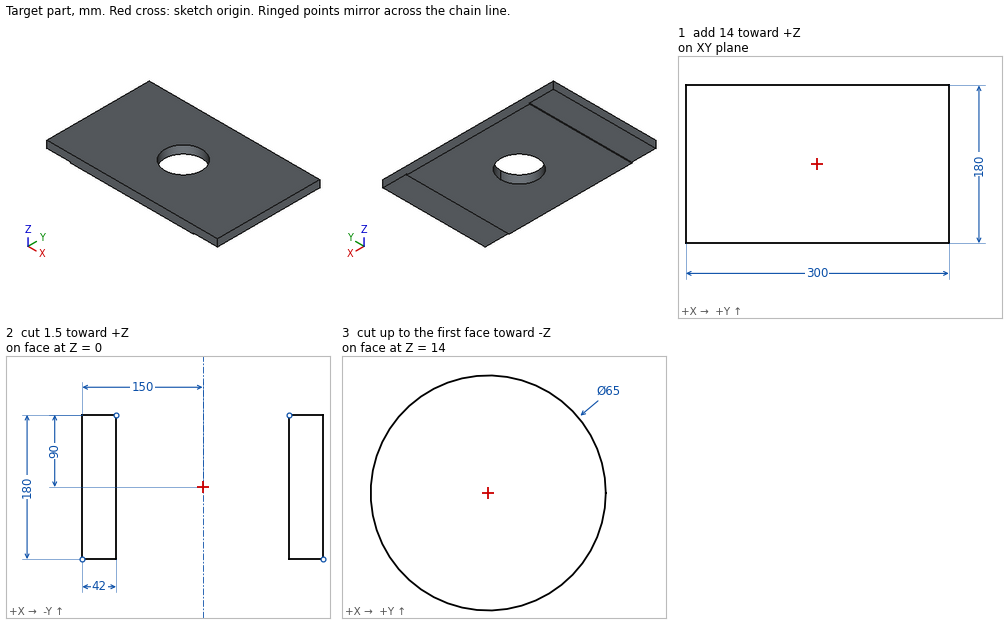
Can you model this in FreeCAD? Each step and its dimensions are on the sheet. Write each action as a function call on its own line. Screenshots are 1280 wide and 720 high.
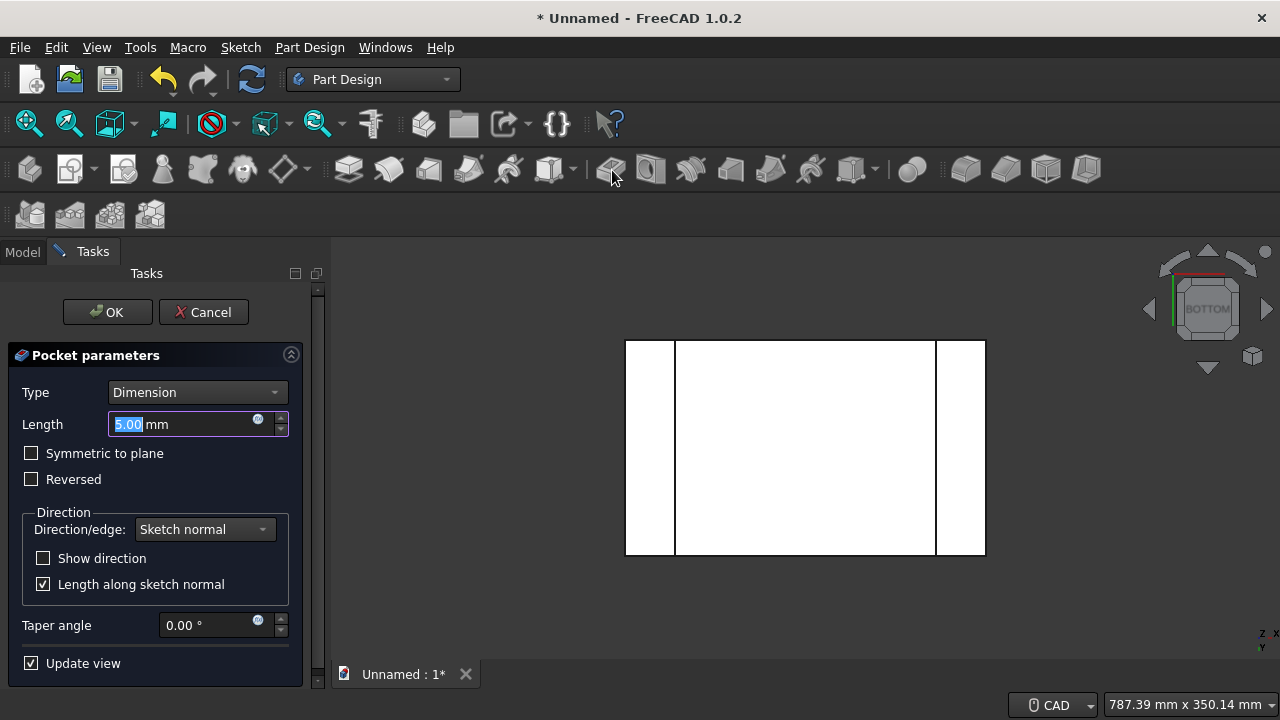
text(1.5)
key(Tab)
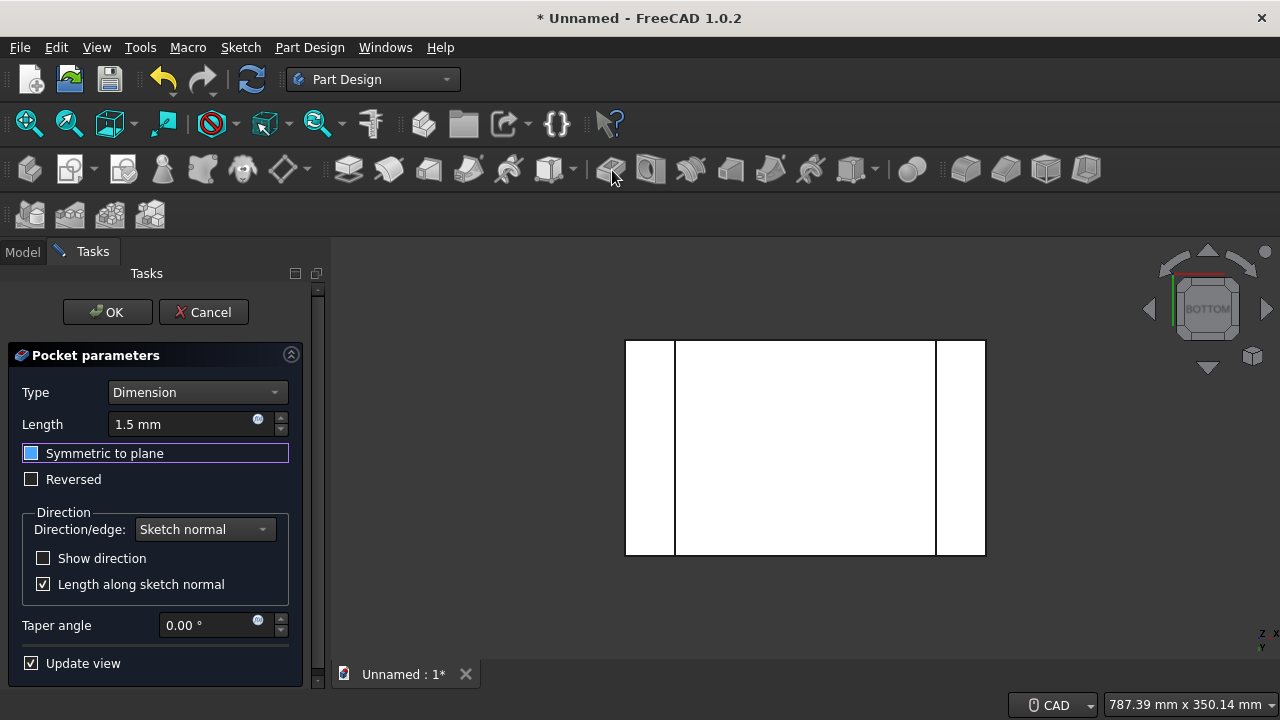
click(108, 312)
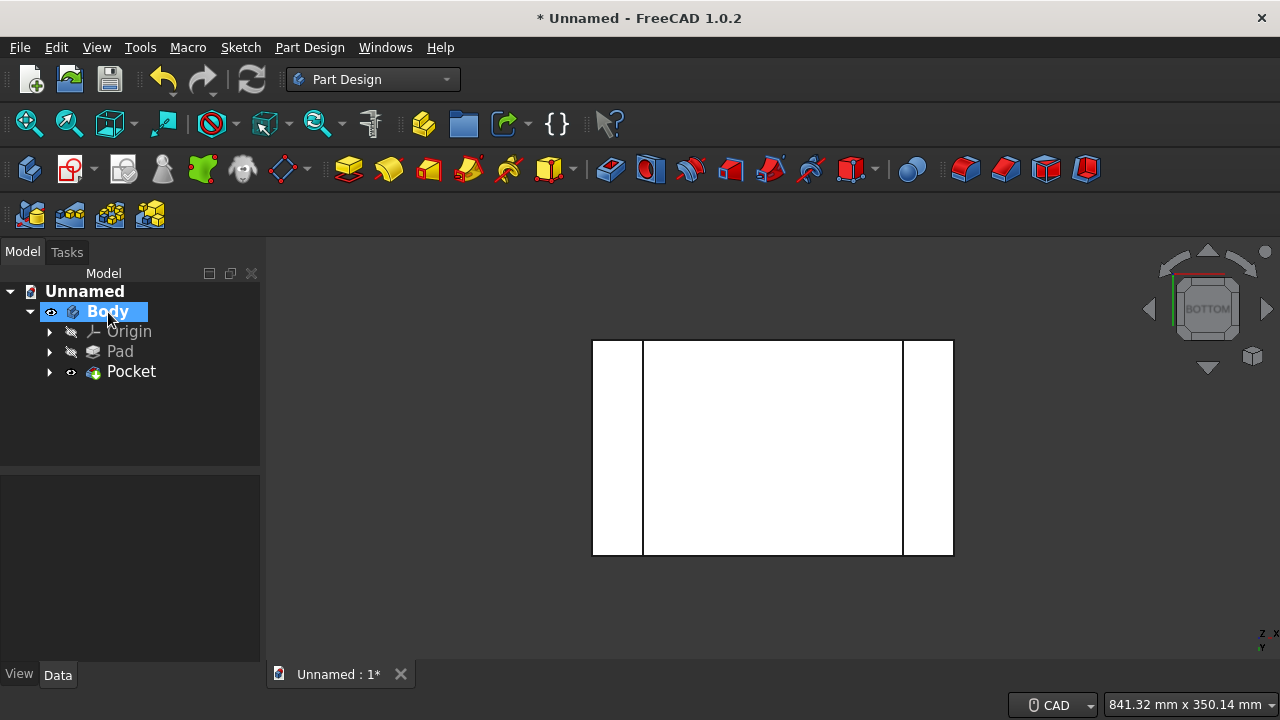
key(0)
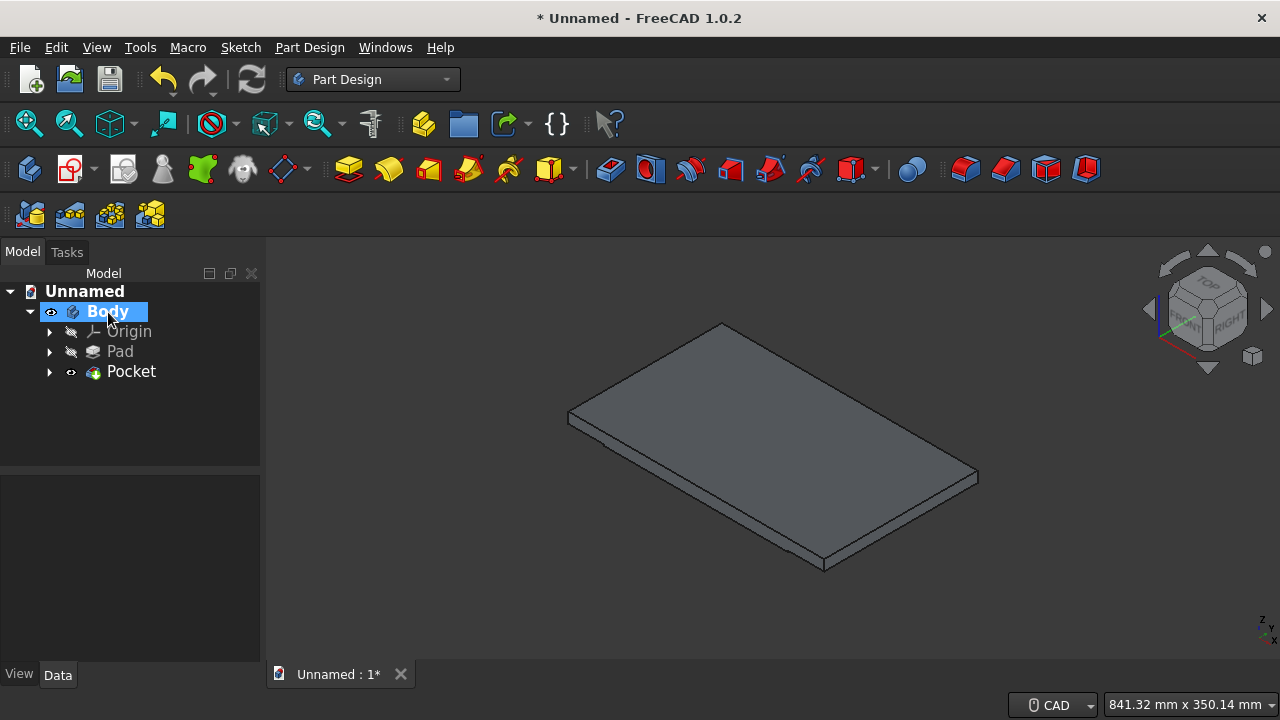
click(810, 461)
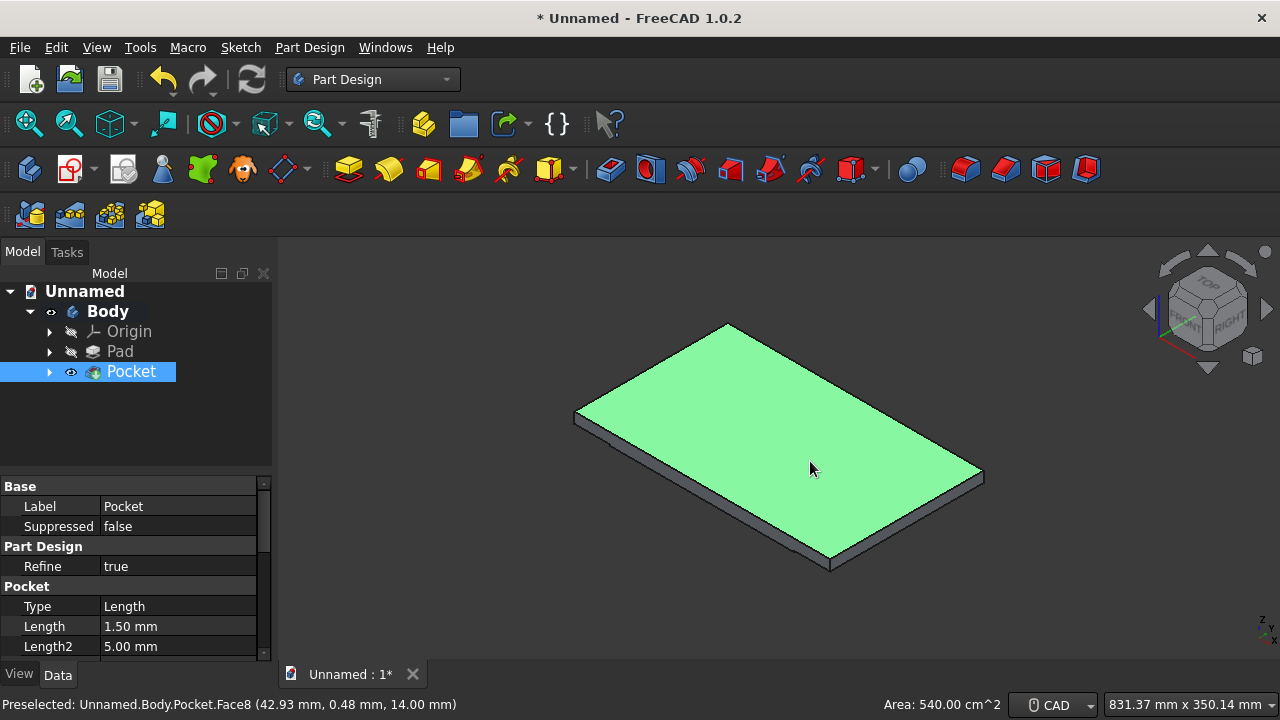
click(70, 170)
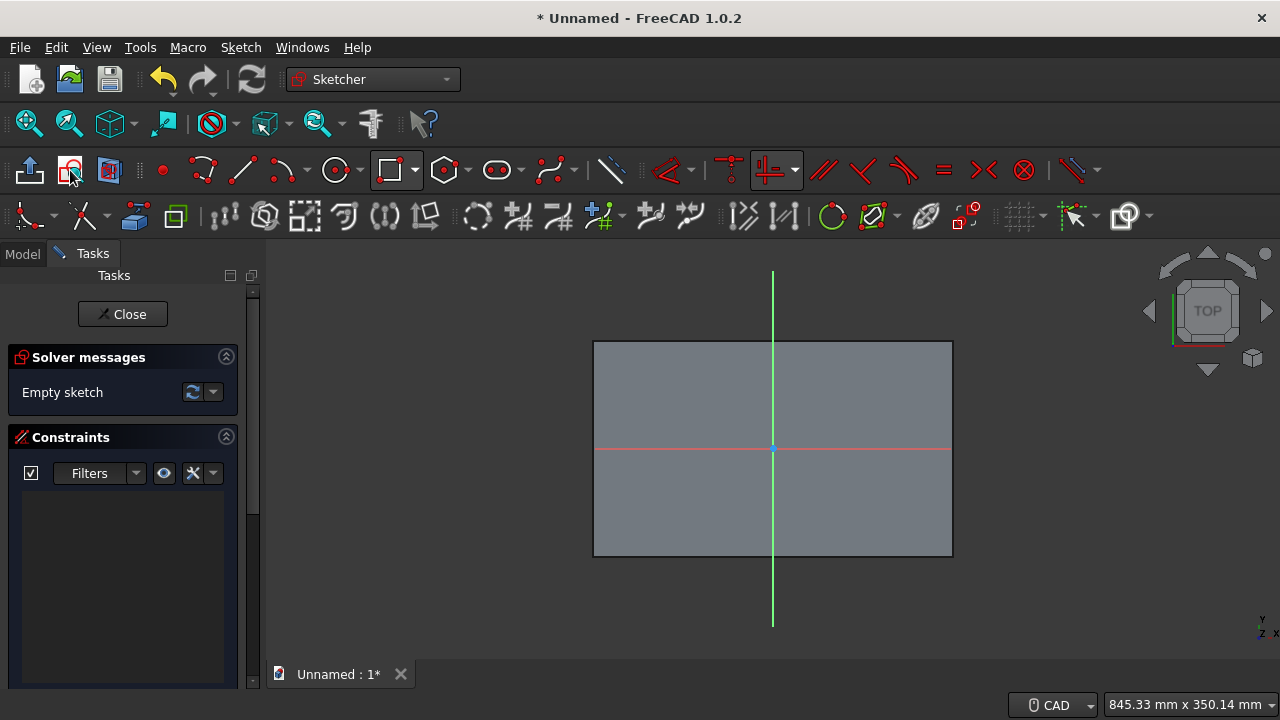
scroll(803, 449, up, 6)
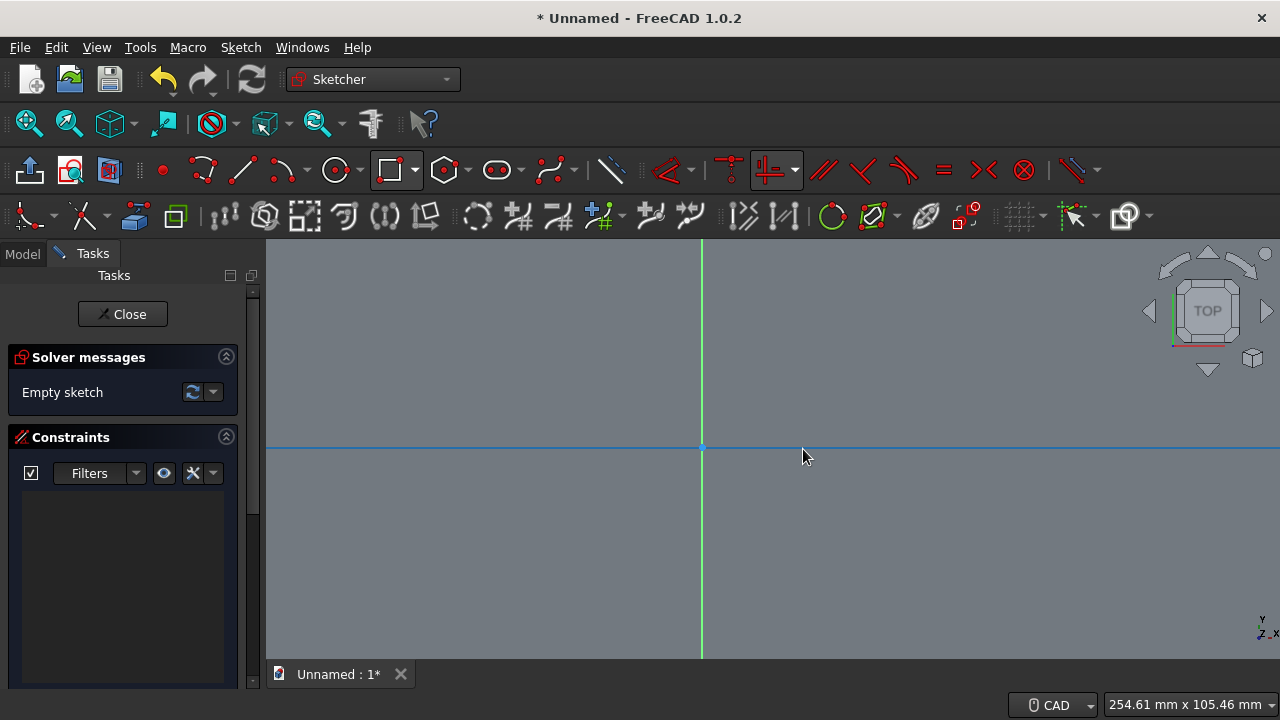
click(336, 170)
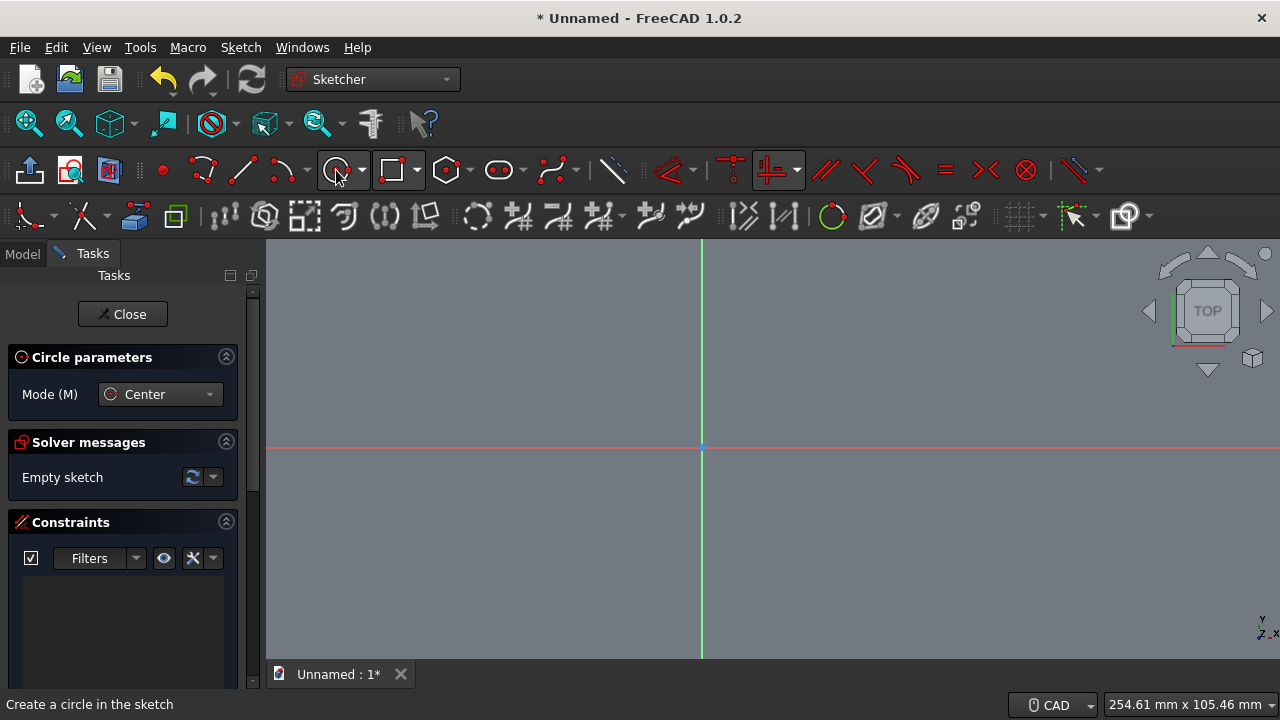
click(702, 448)
click(794, 356)
key(Escape)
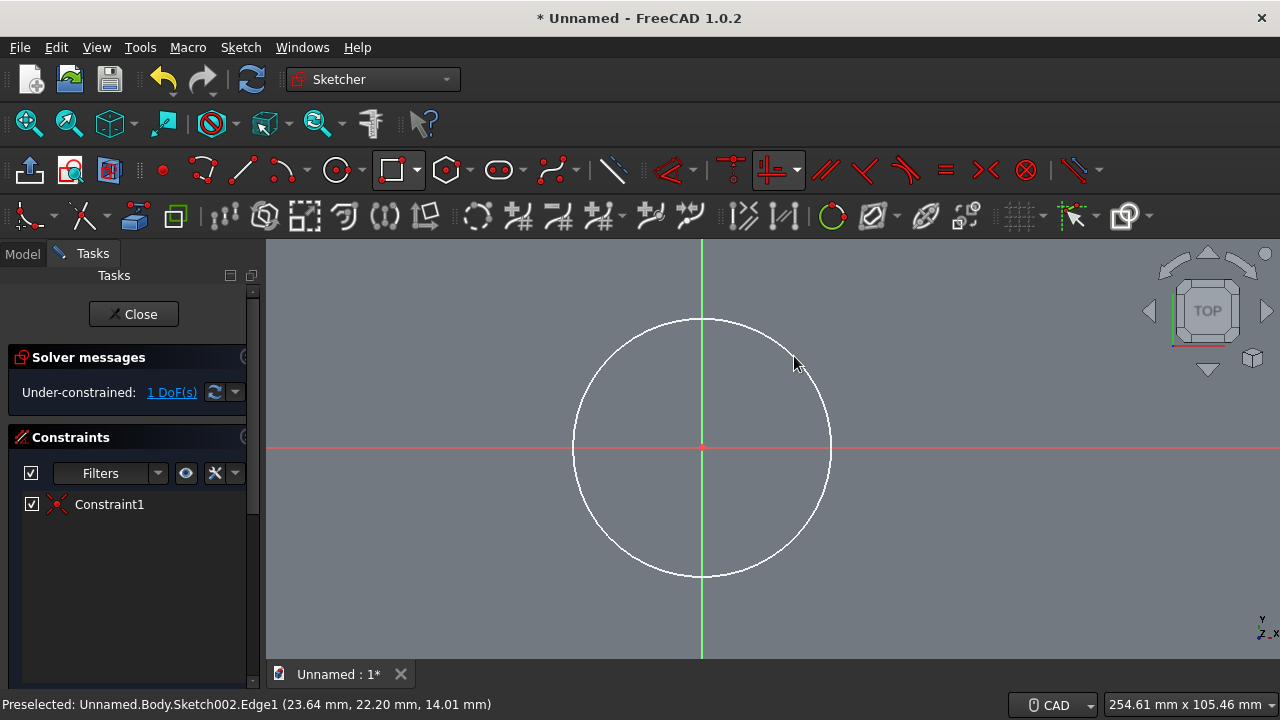
click(668, 170)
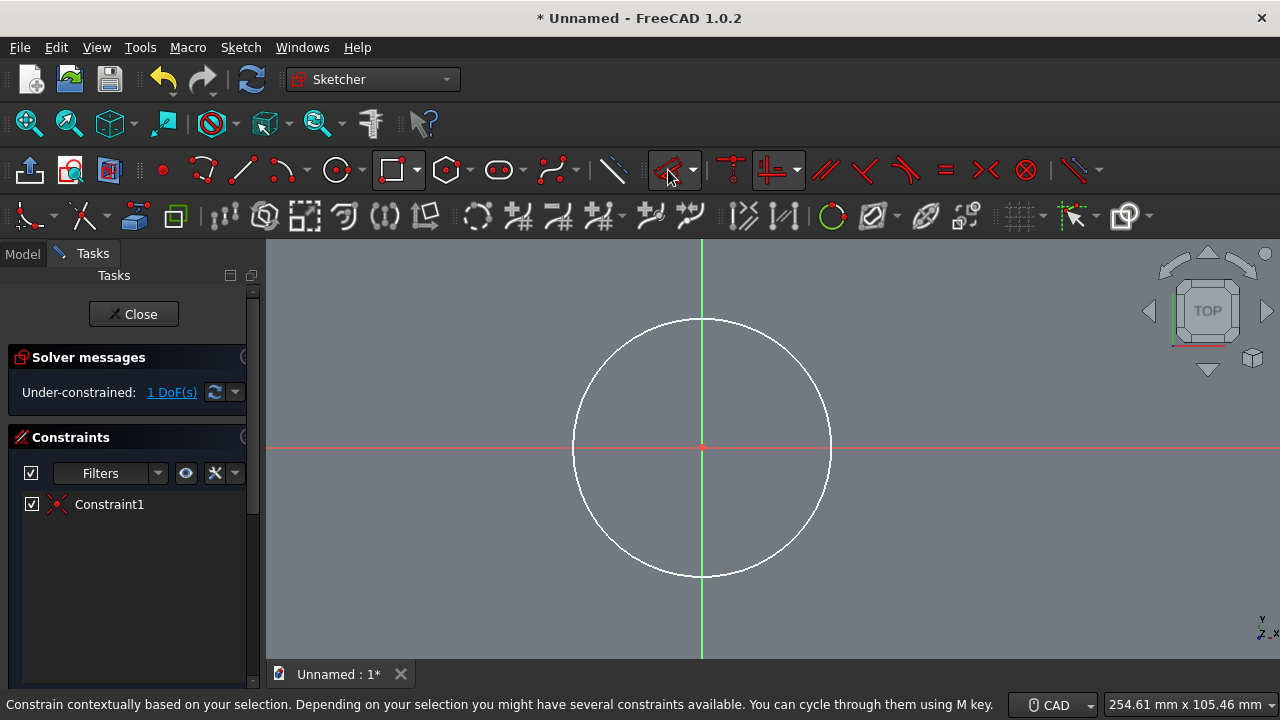
click(793, 356)
click(816, 333)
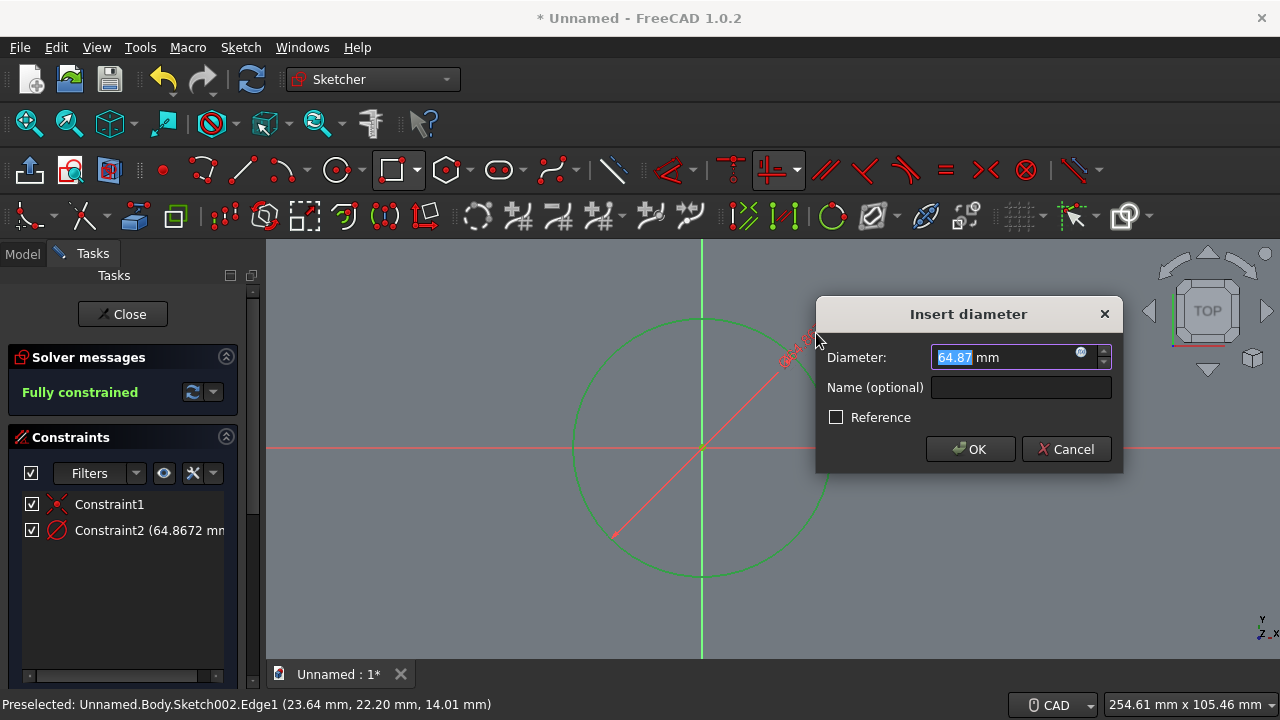
text(65)
key(Return)
key(Escape)